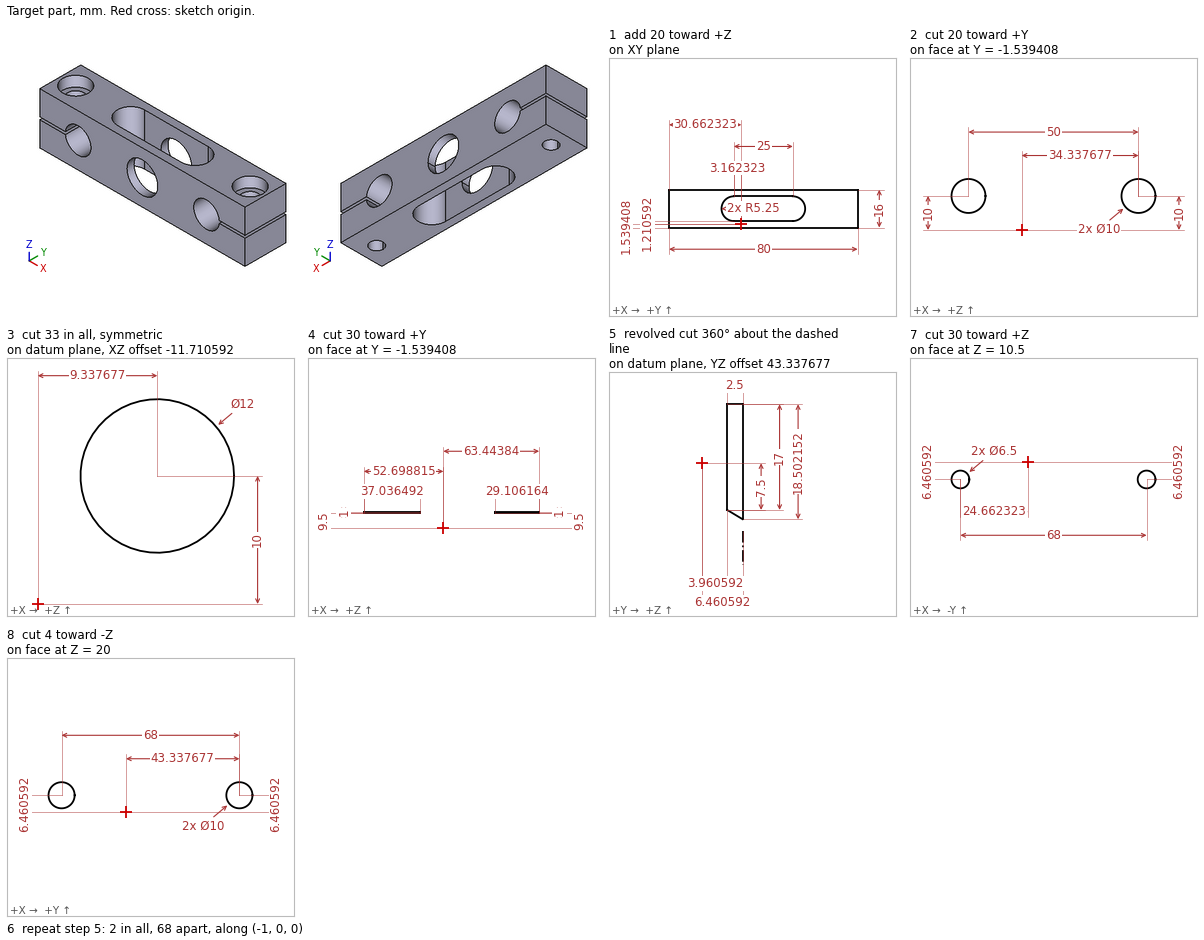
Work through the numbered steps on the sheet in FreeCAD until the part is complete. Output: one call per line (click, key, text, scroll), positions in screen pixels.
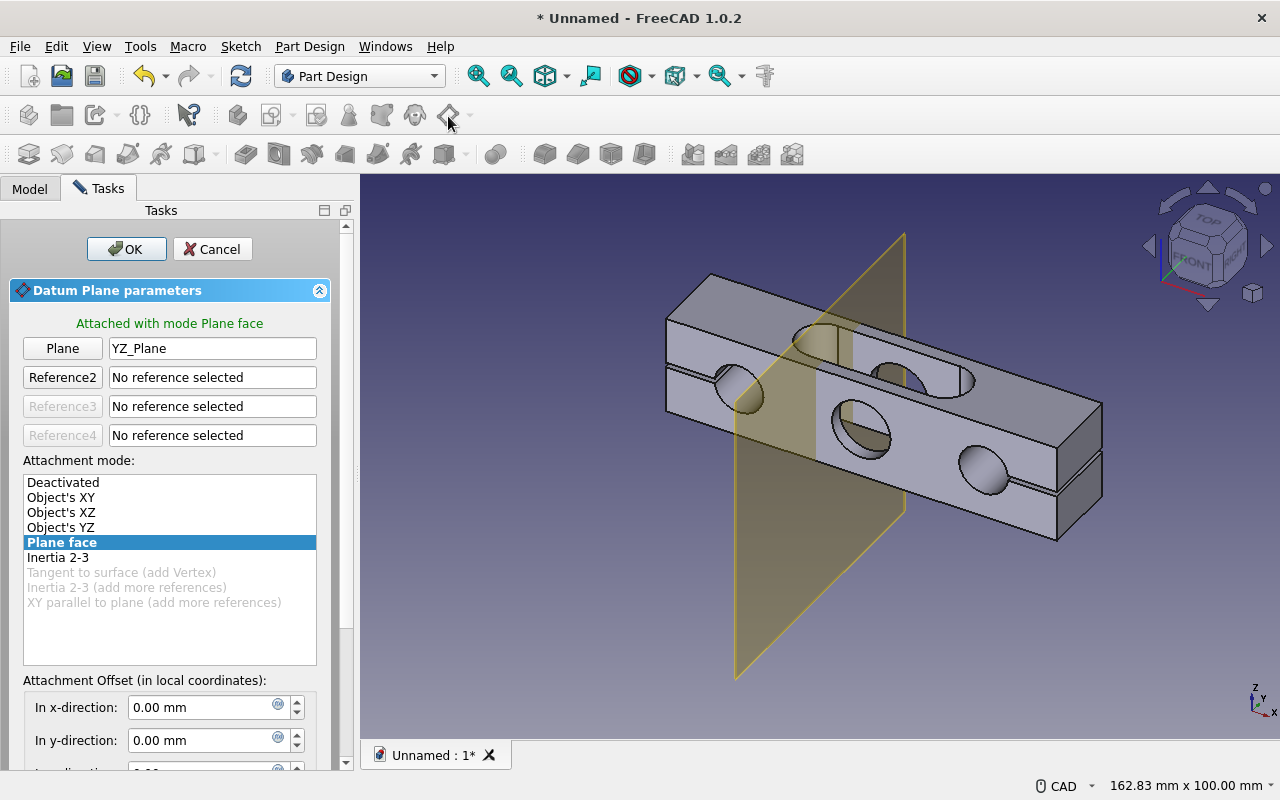
scroll(346, 495, down, 2)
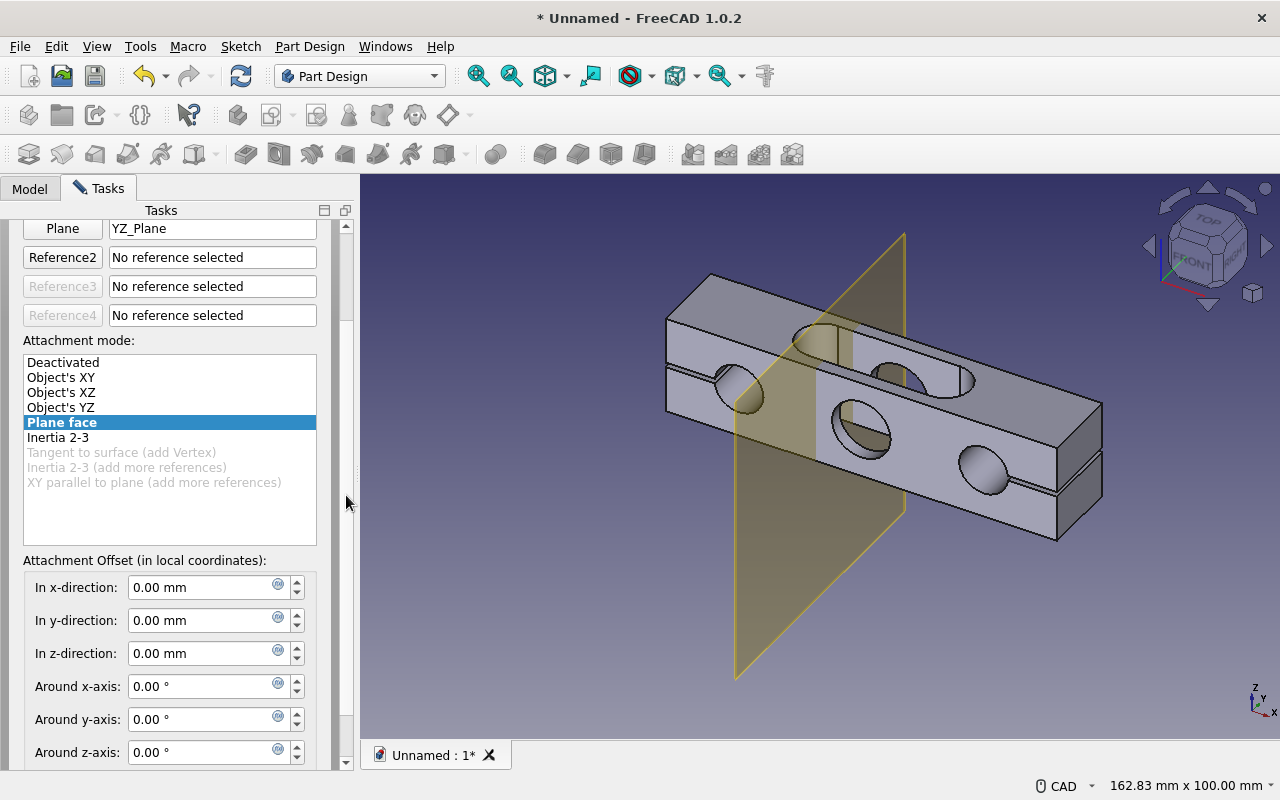
triple_click(210, 654)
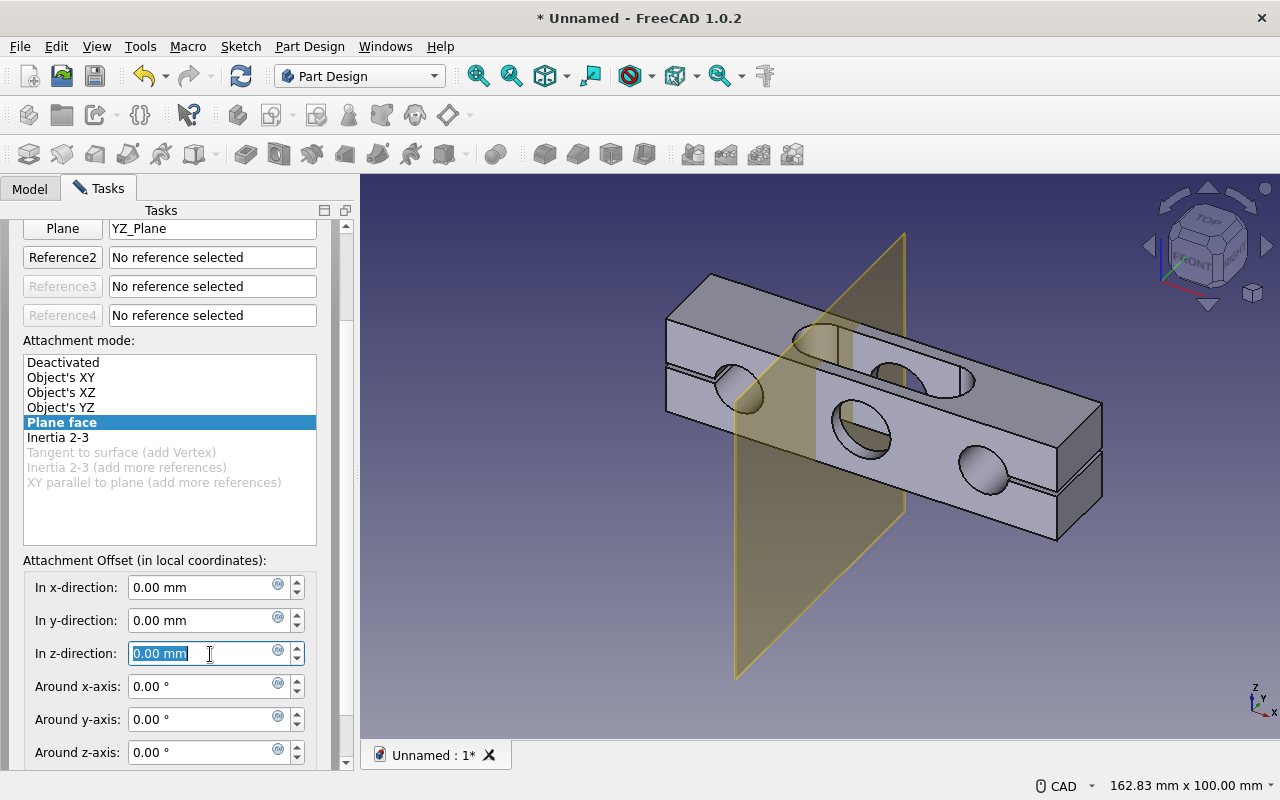
text(43.337677)
key(Tab)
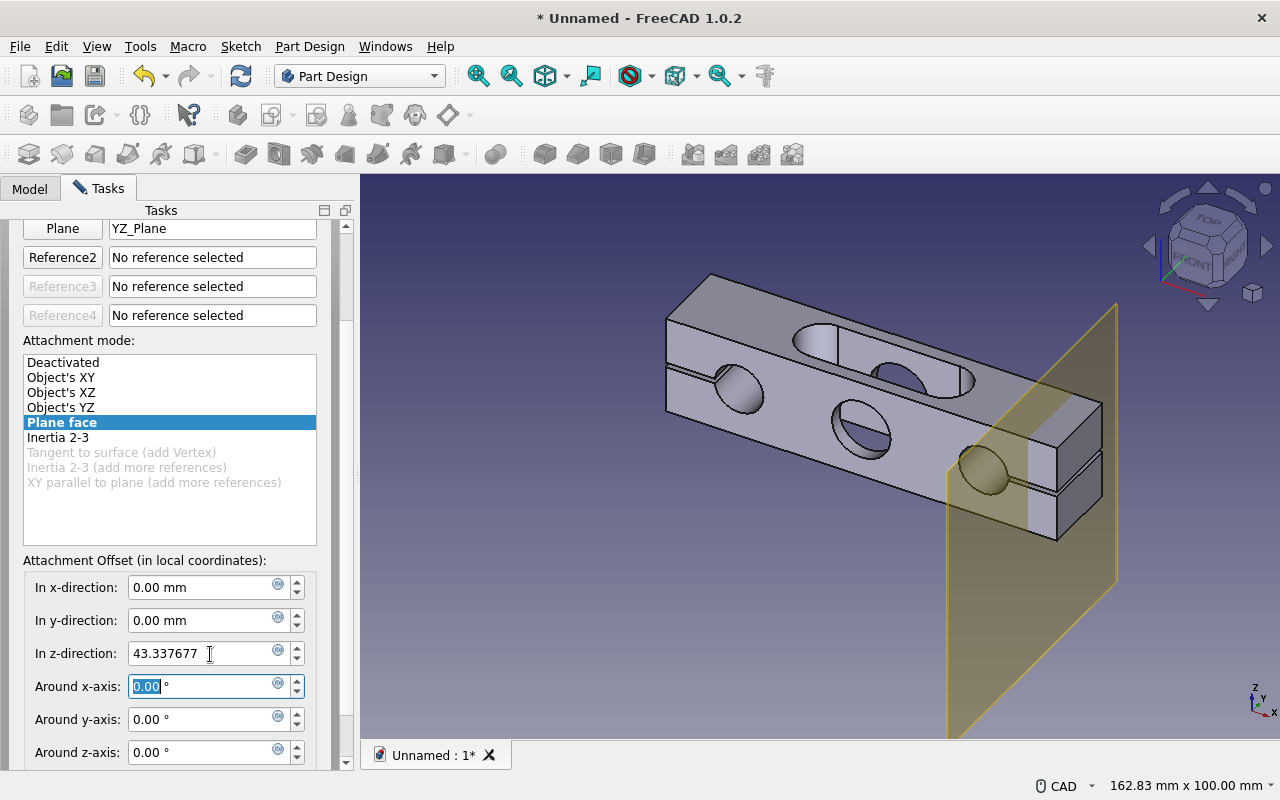
scroll(346, 495, up, 3)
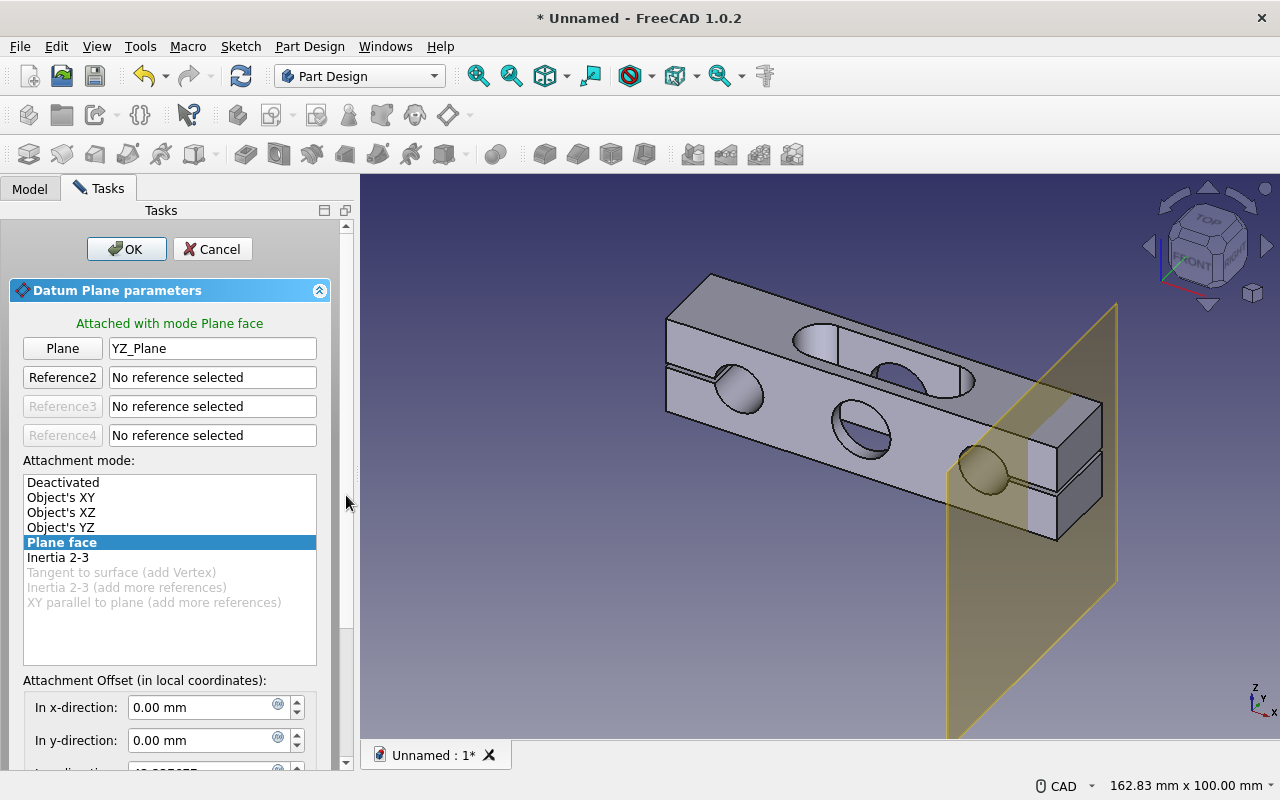
click(127, 249)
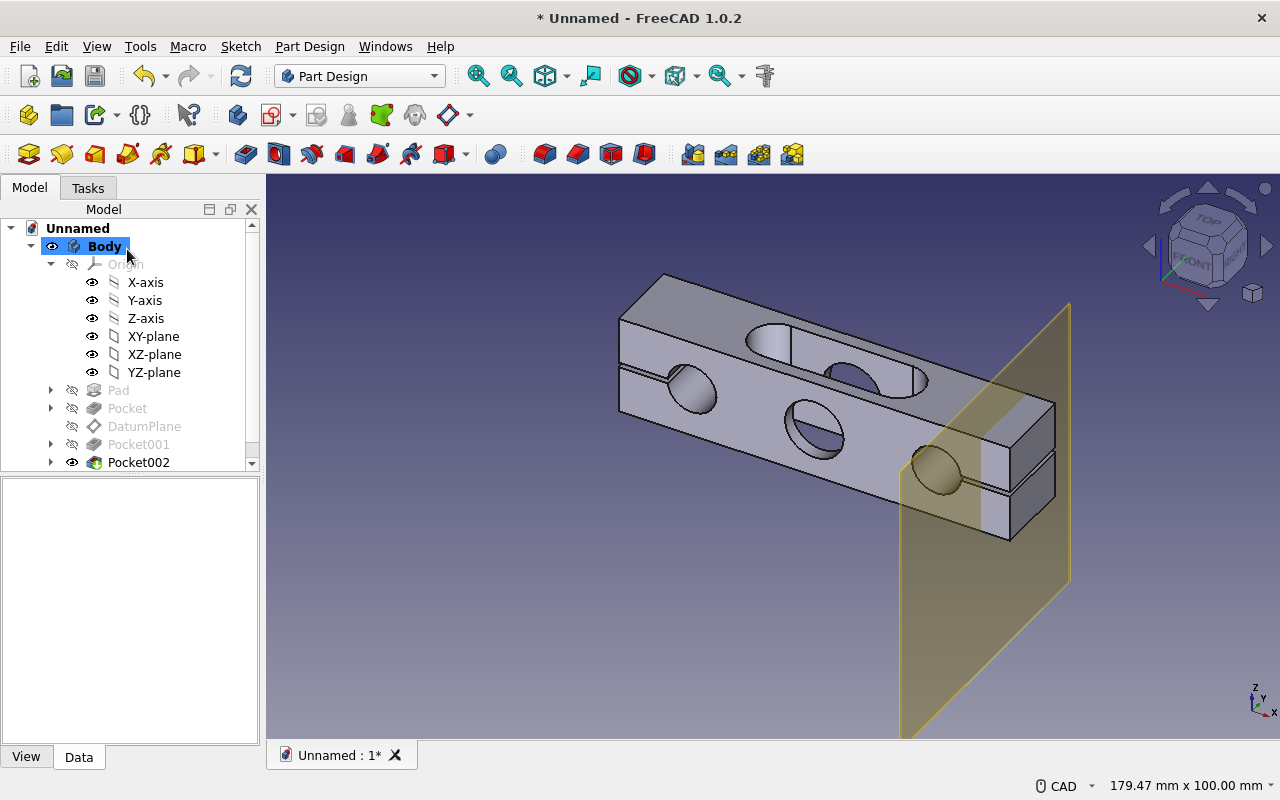
scroll(101, 350, down, 3)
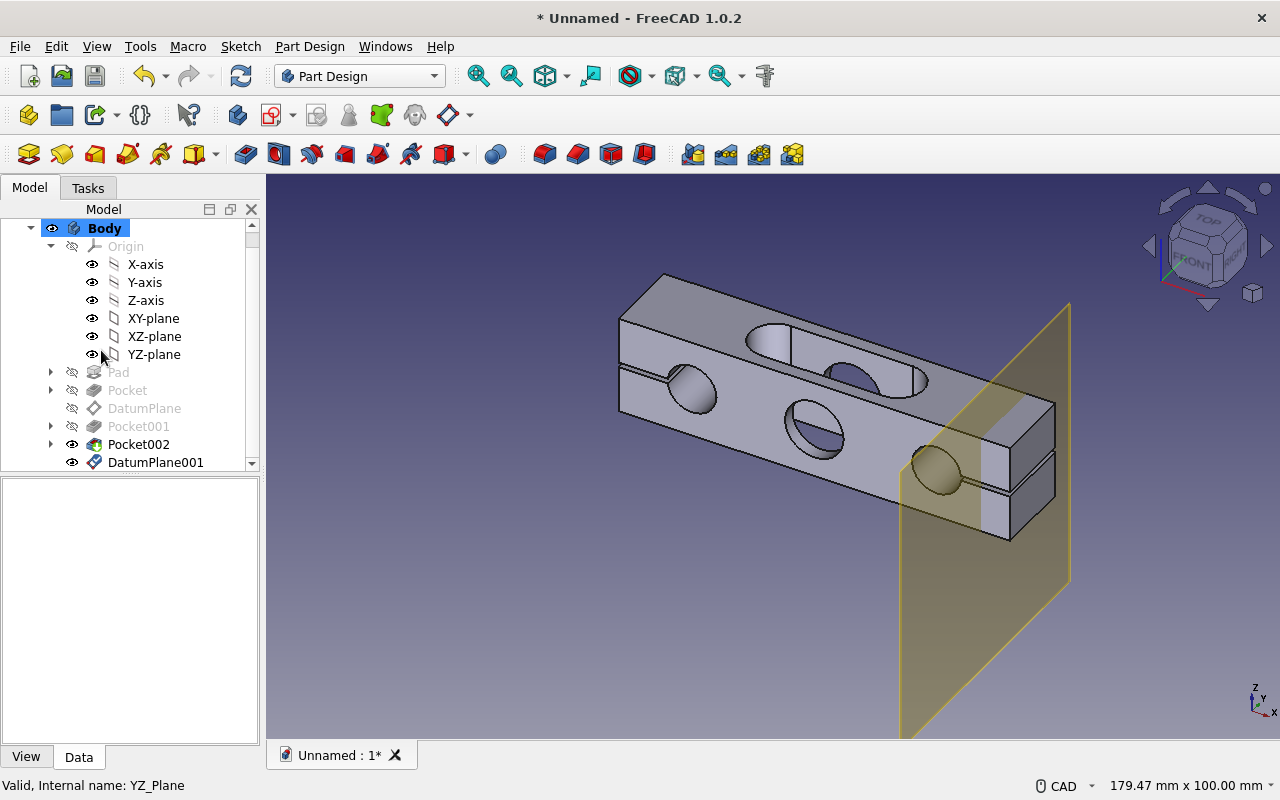
click(117, 462)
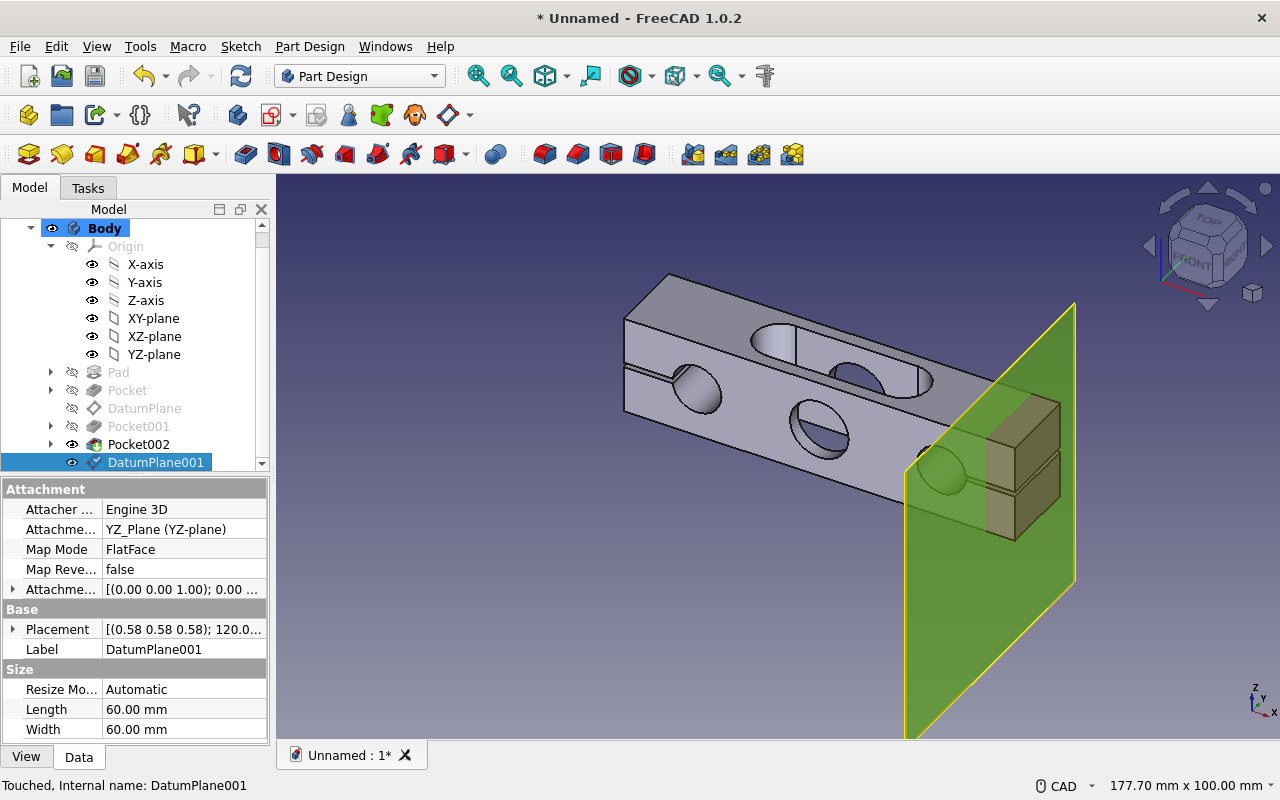
click(270, 116)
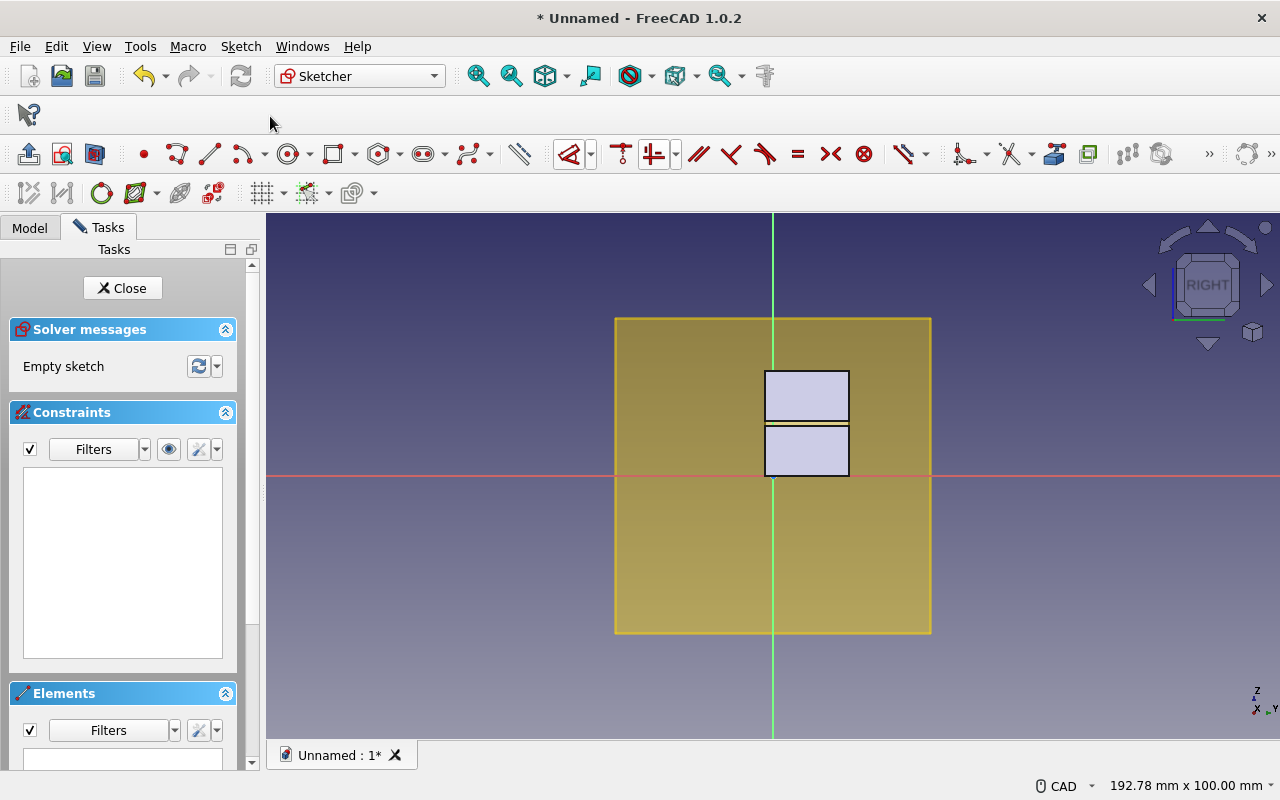
click(95, 154)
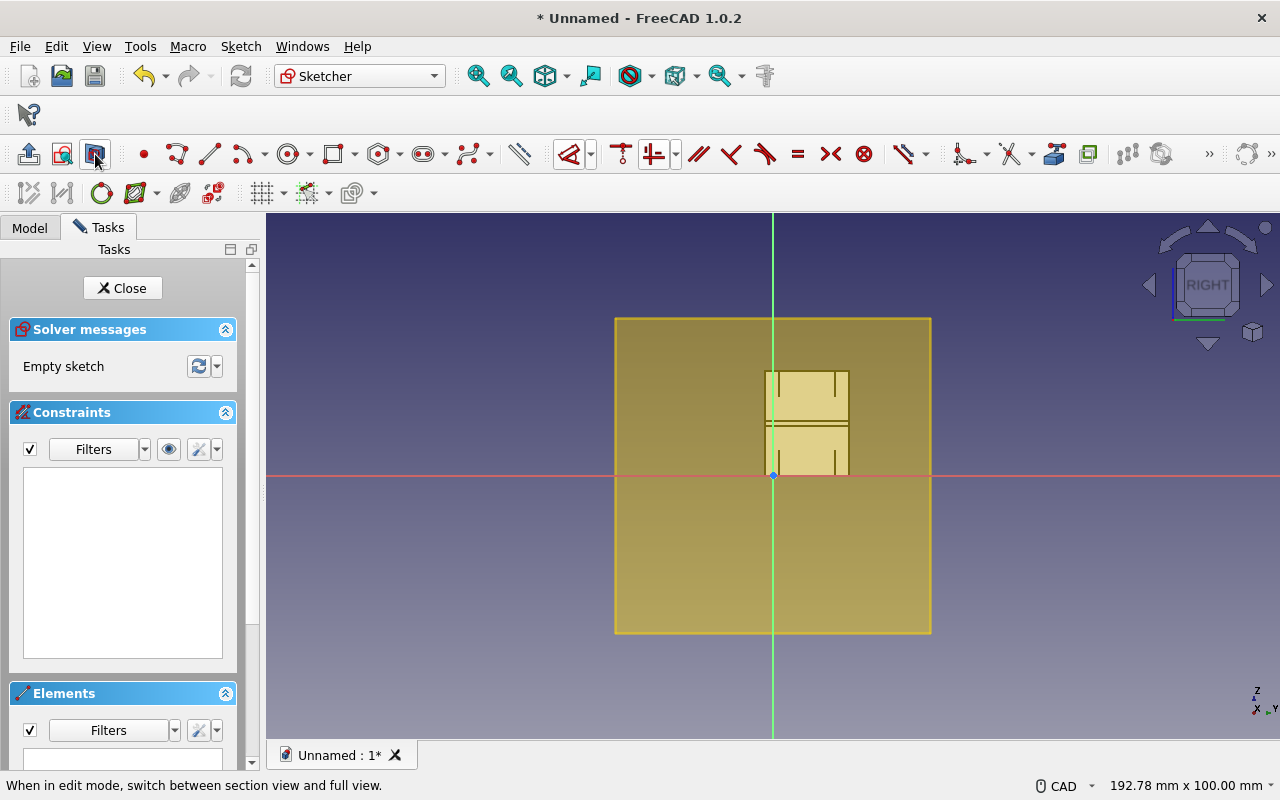
scroll(860, 509, up, 4)